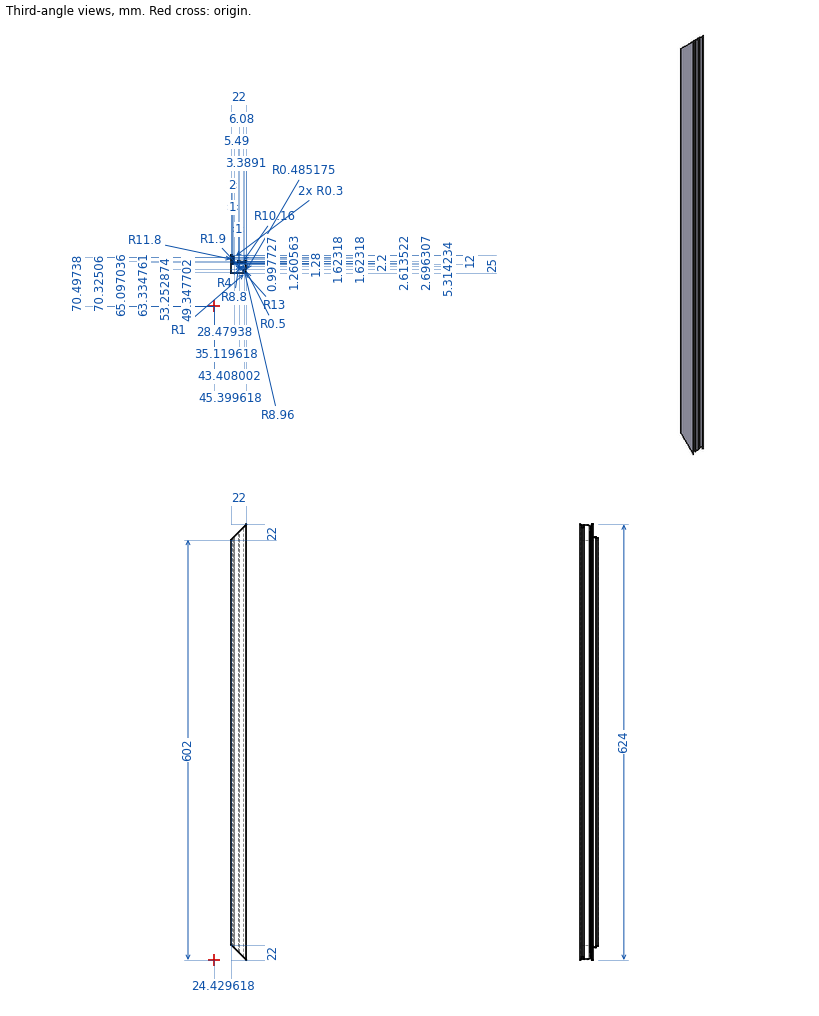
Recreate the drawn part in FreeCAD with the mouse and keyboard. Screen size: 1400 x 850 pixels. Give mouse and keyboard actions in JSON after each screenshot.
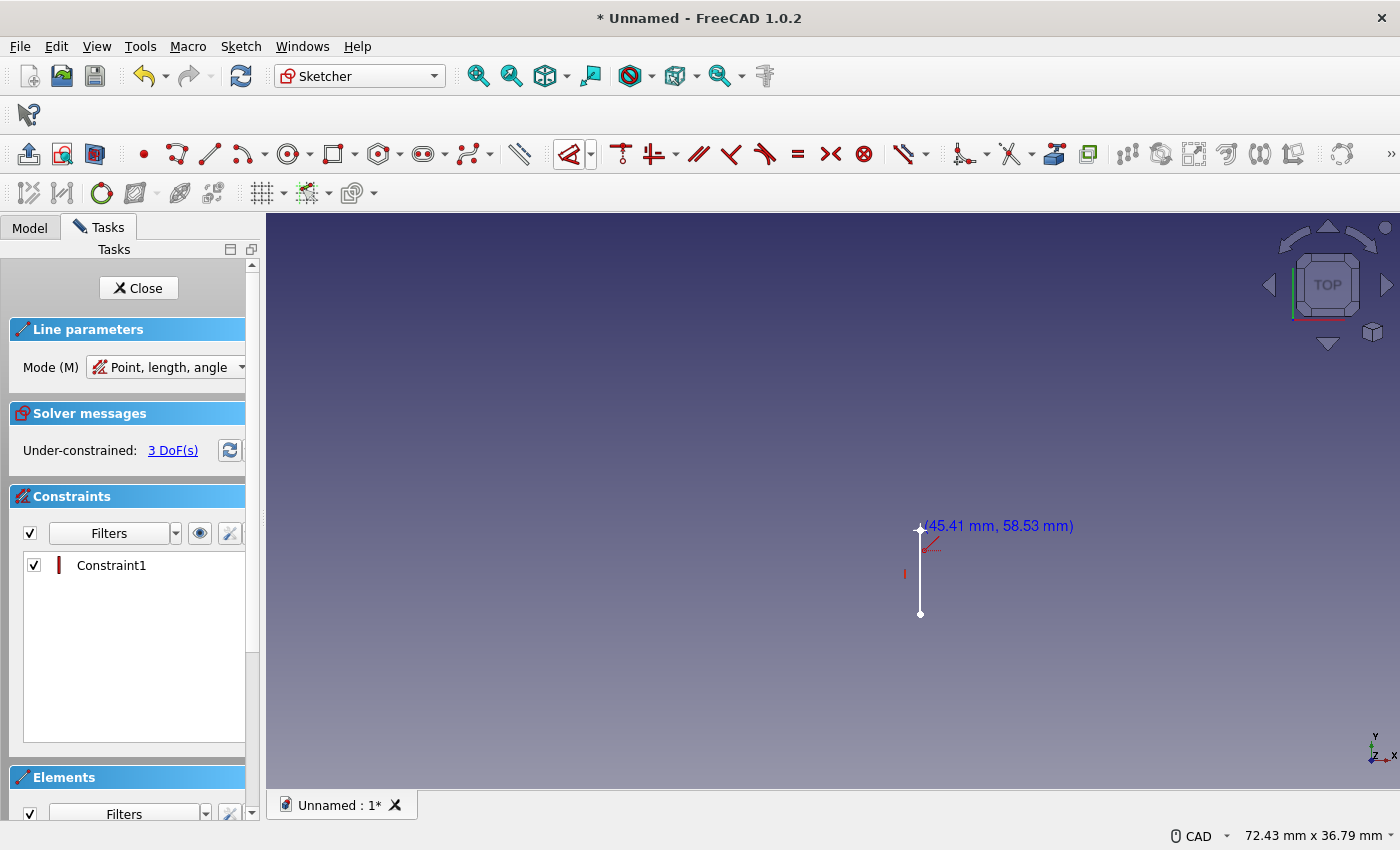
{"action": "key", "text": "g m"}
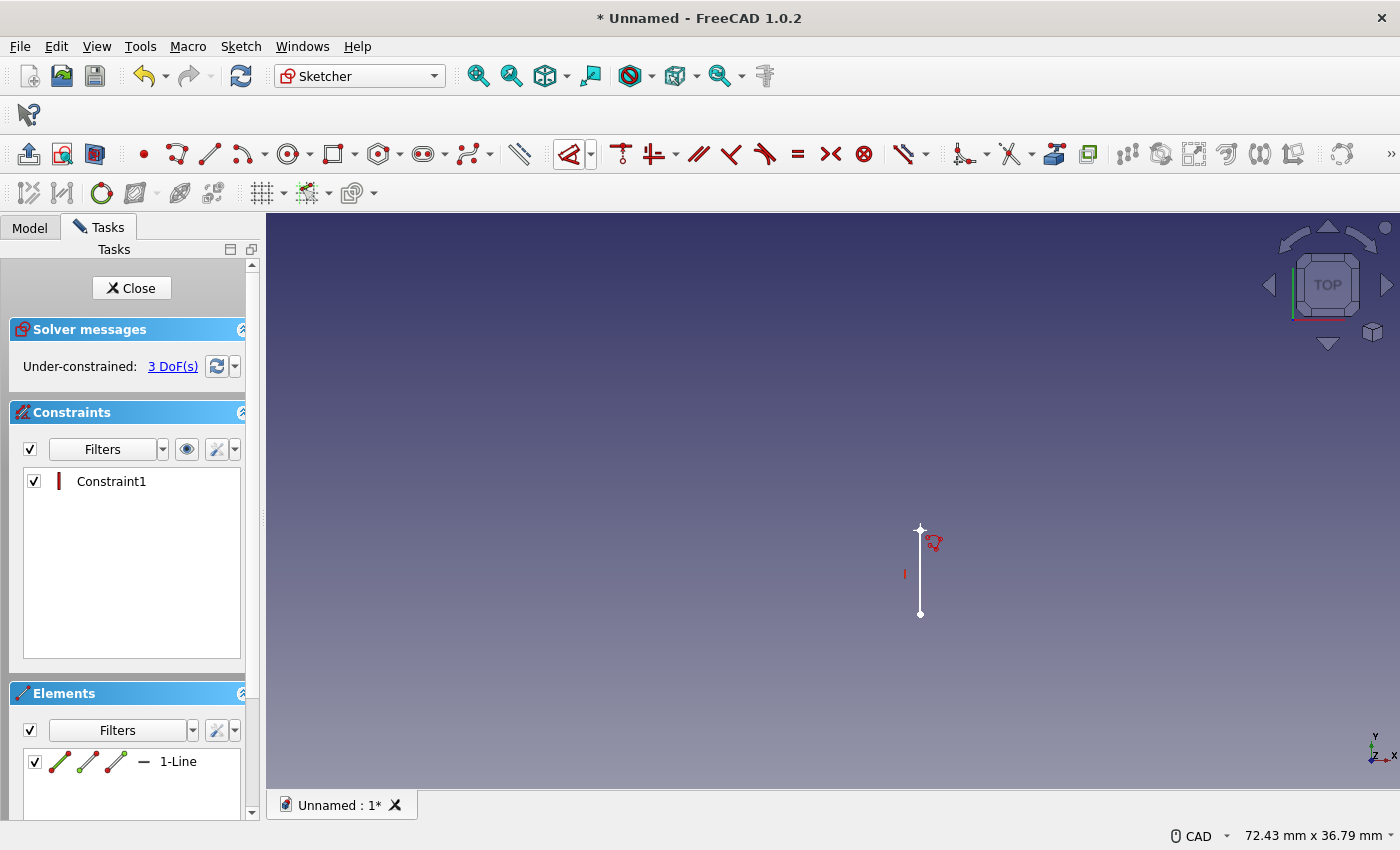
{"action": "left_click", "coordinate": [857, 468]}
{"action": "left_click", "coordinate": [762, 468]}
{"action": "left_click", "coordinate": [762, 452]}
{"action": "right_click", "coordinate": [762, 452]}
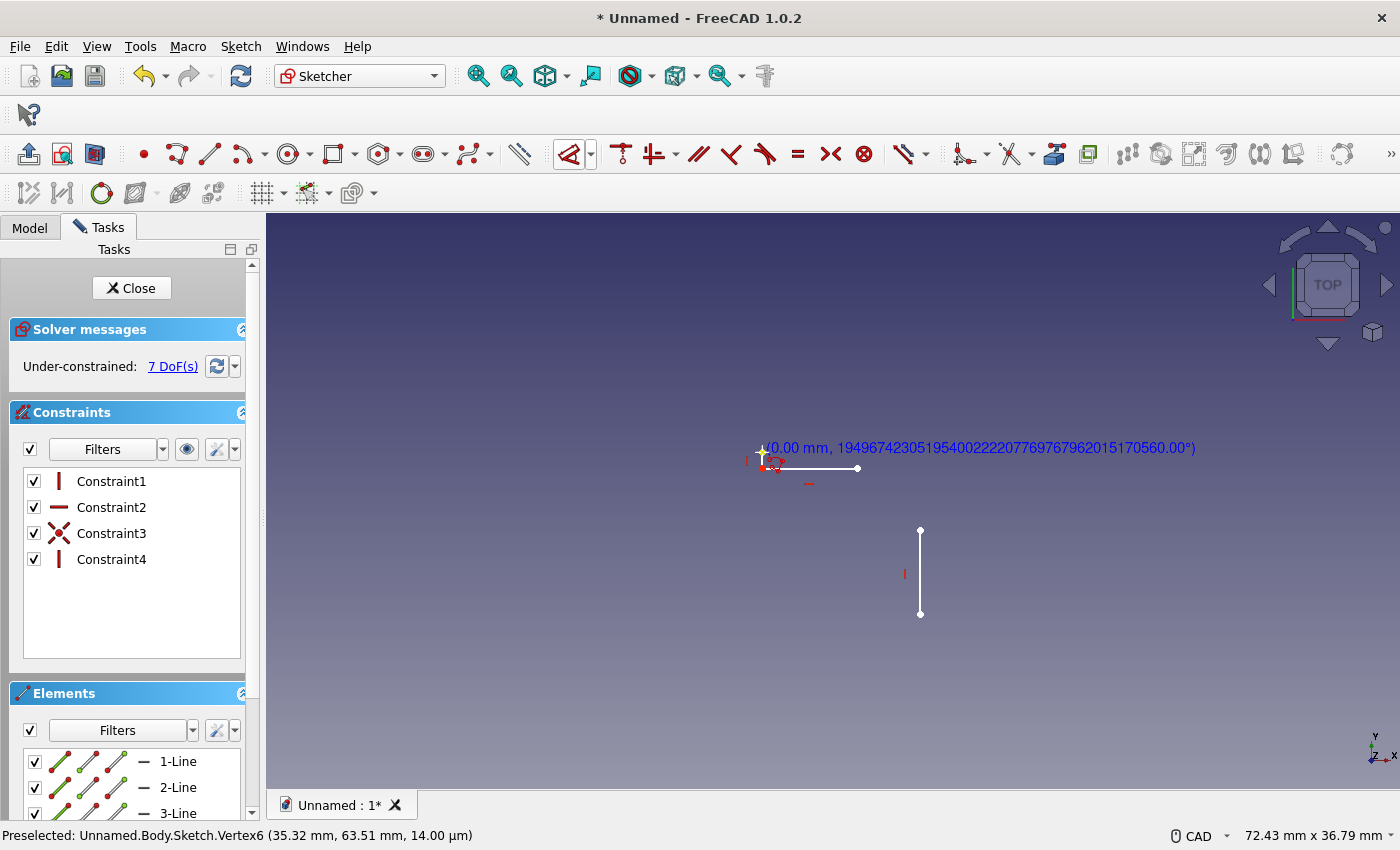
{"action": "left_click", "coordinate": [889, 456]}
{"action": "left_click", "coordinate": [936, 440]}
{"action": "left_click", "coordinate": [936, 421]}
{"action": "left_click", "coordinate": [883, 438]}
{"action": "right_click", "coordinate": [883, 438]}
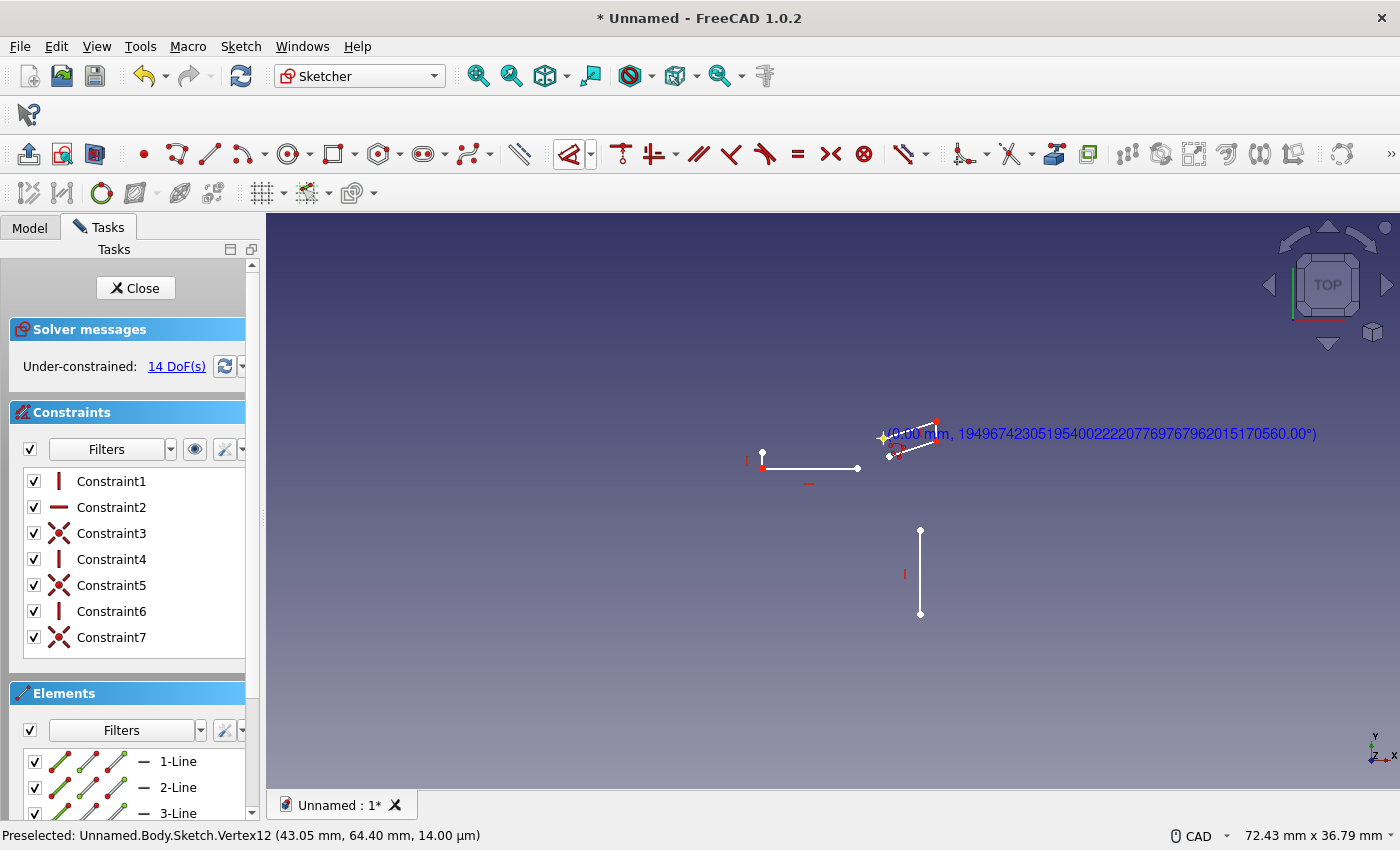
{"action": "left_click", "coordinate": [759, 433]}
{"action": "left_click", "coordinate": [743, 433]}
{"action": "left_click", "coordinate": [743, 468]}
{"action": "left_click", "coordinate": [657, 468]}
{"action": "left_click", "coordinate": [651, 426]}
{"action": "right_click", "coordinate": [651, 426]}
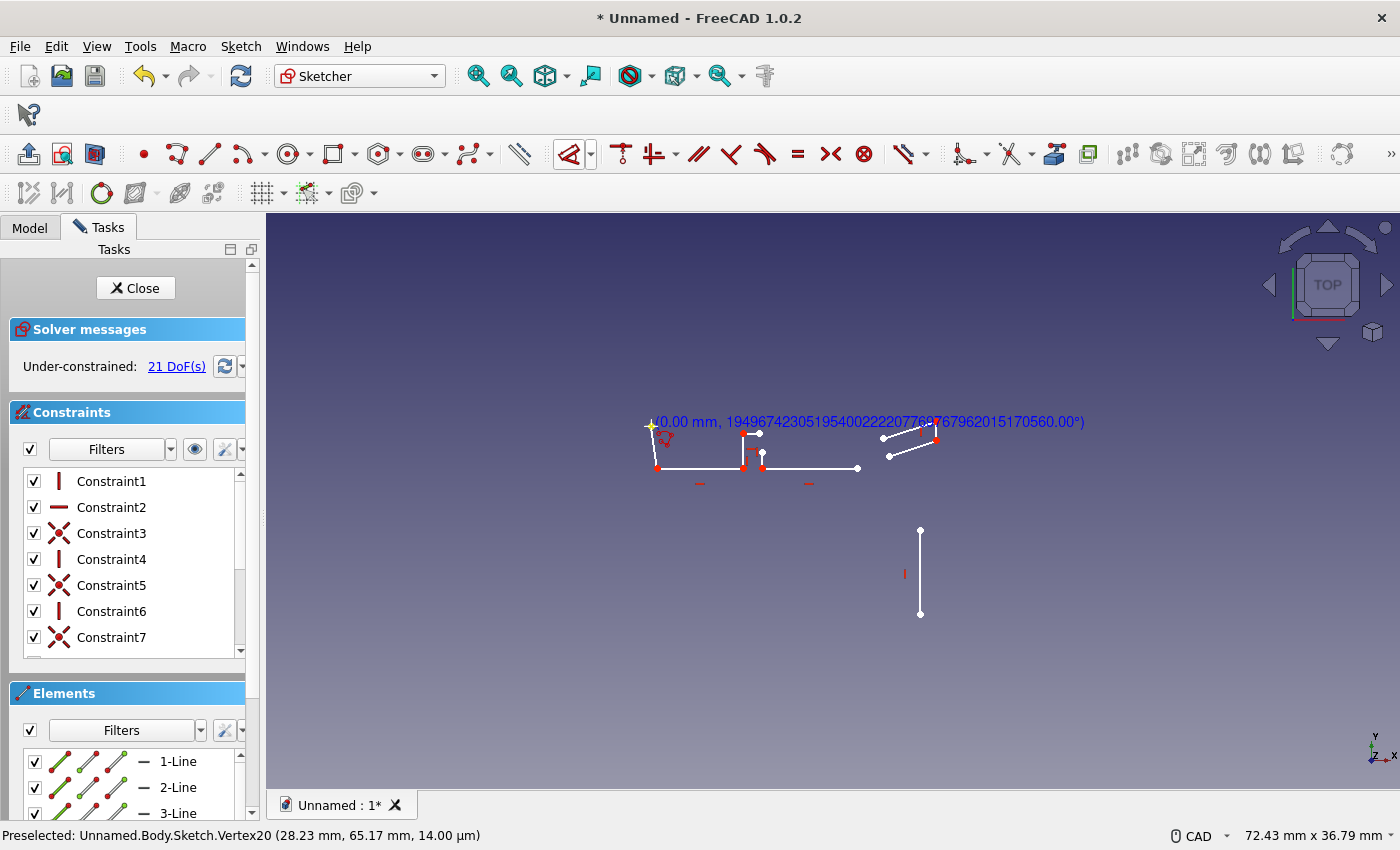
{"action": "key", "text": "g l"}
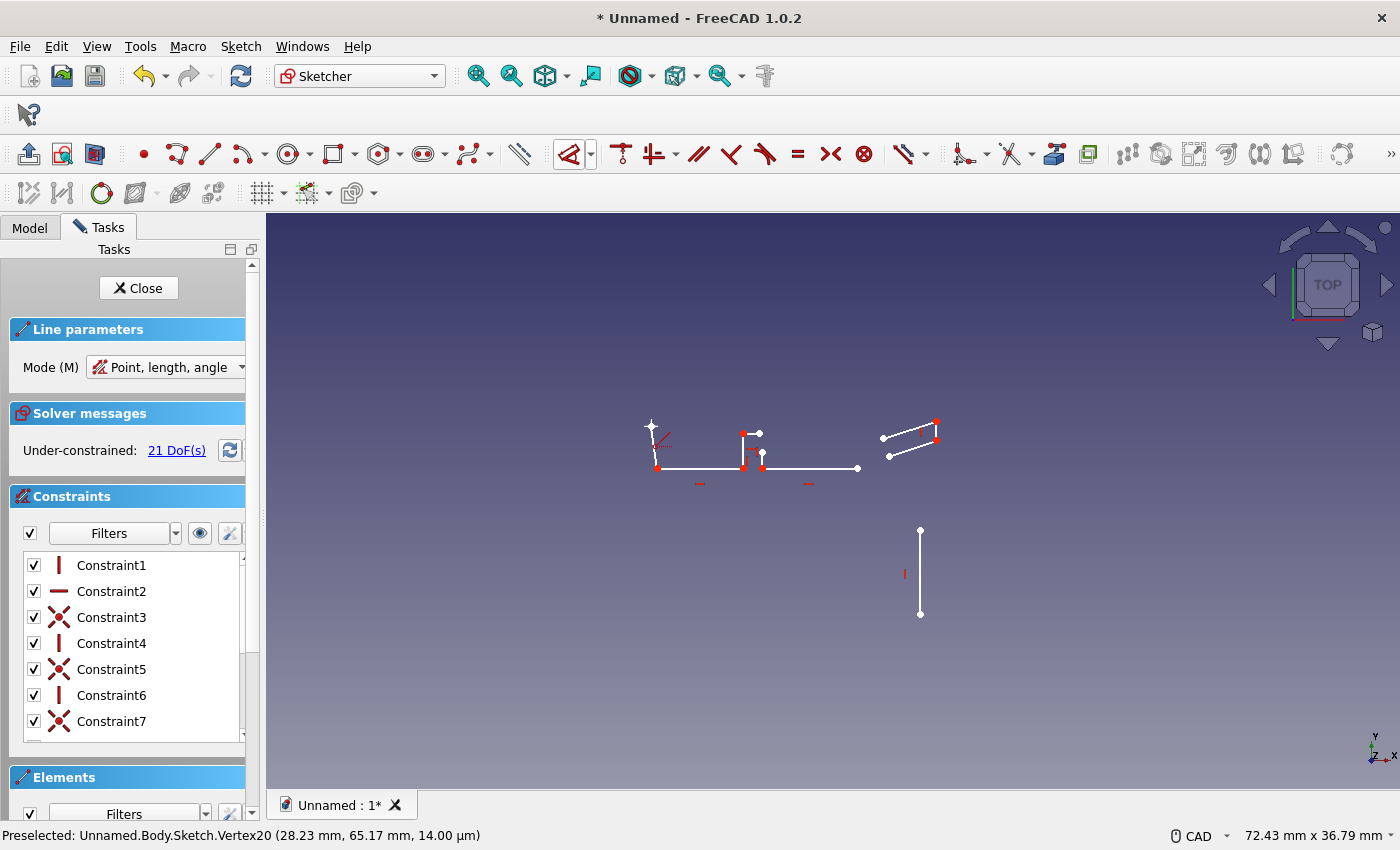
{"action": "left_click", "coordinate": [651, 374]}
{"action": "left_click", "coordinate": [655, 349]}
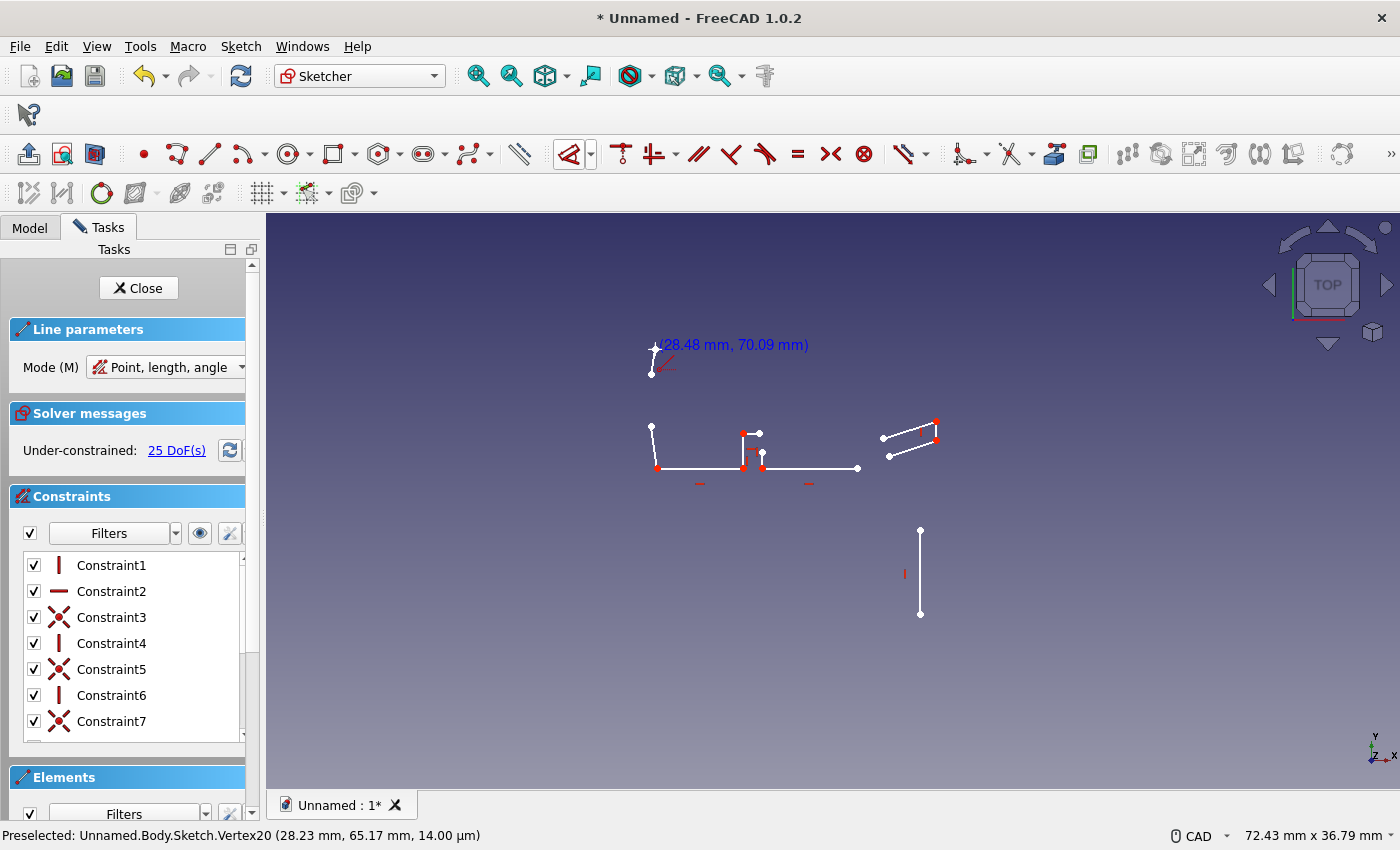
{"action": "scroll", "coordinate": [651, 344], "scroll_direction": "up", "scroll_amount": 5}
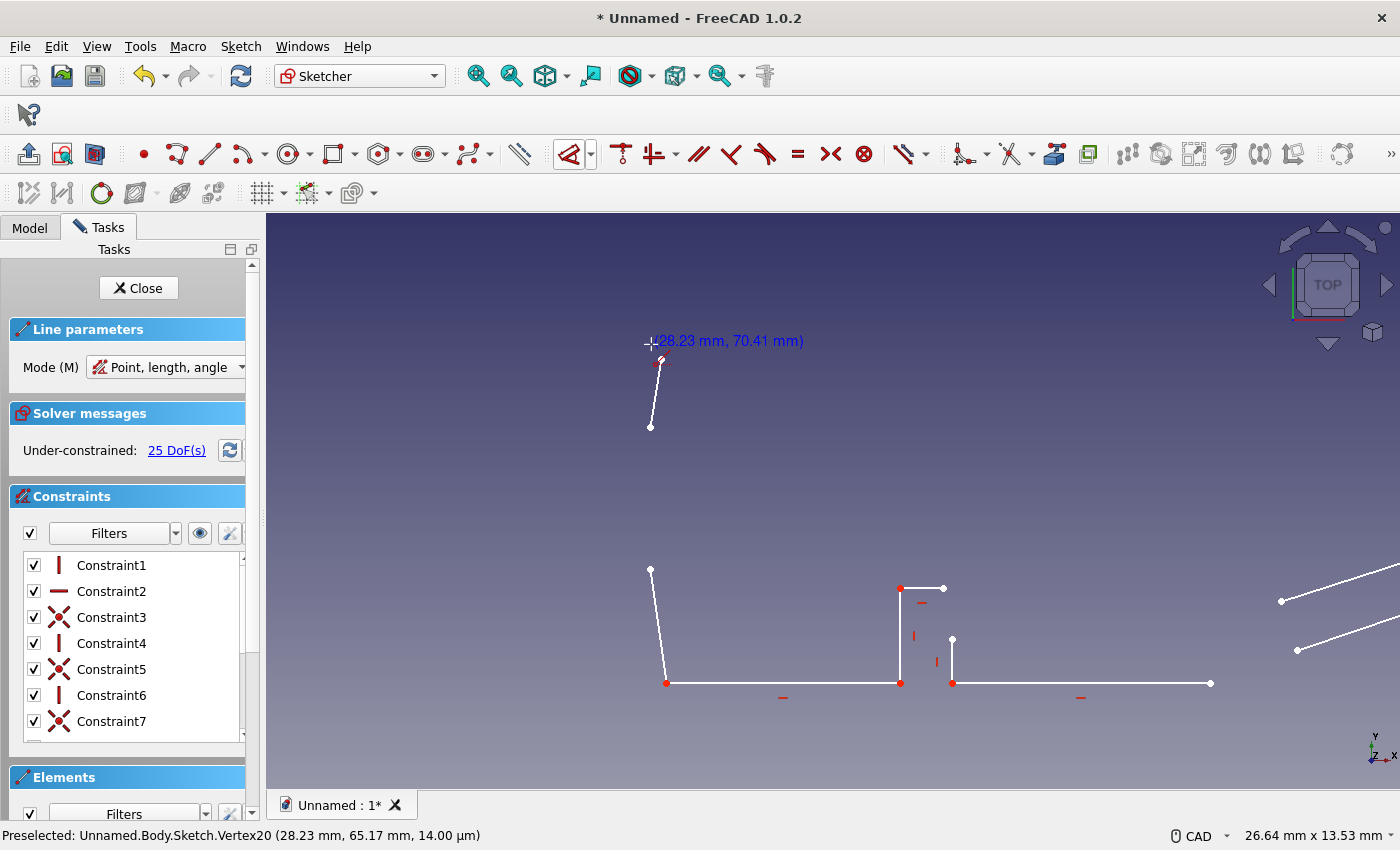
{"action": "left_click", "coordinate": [650, 342]}
{"action": "left_click", "coordinate": [625, 339]}